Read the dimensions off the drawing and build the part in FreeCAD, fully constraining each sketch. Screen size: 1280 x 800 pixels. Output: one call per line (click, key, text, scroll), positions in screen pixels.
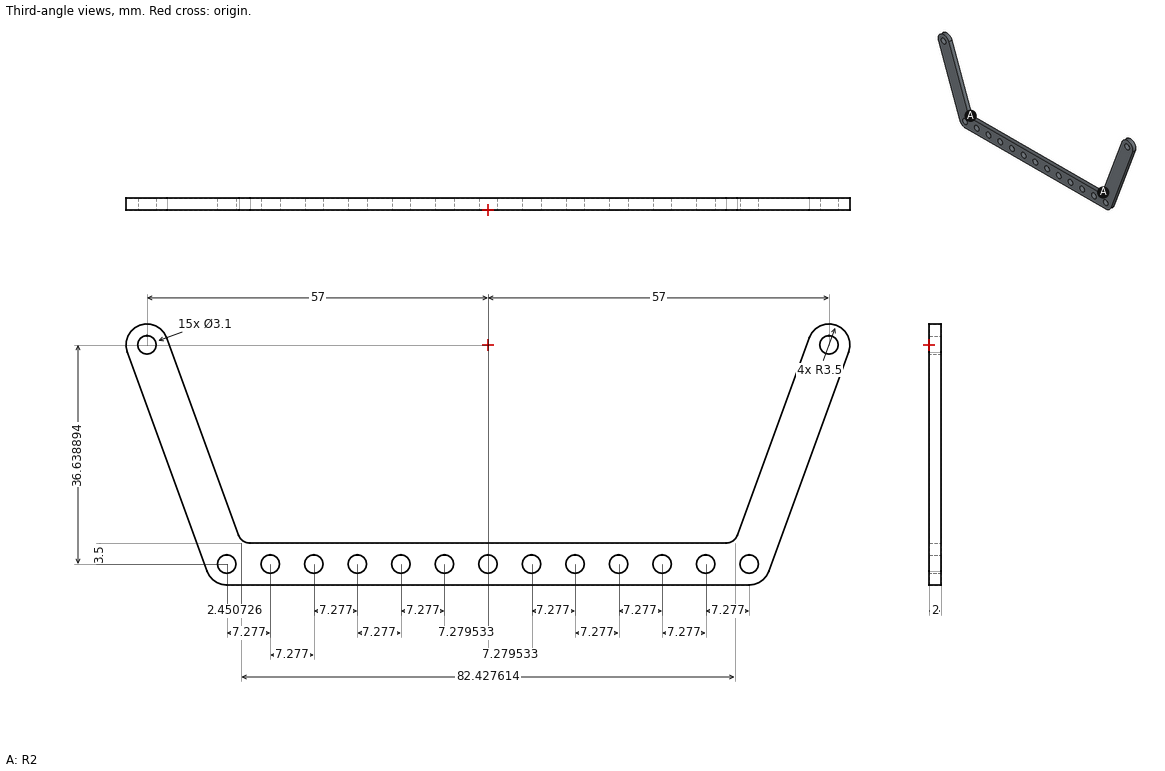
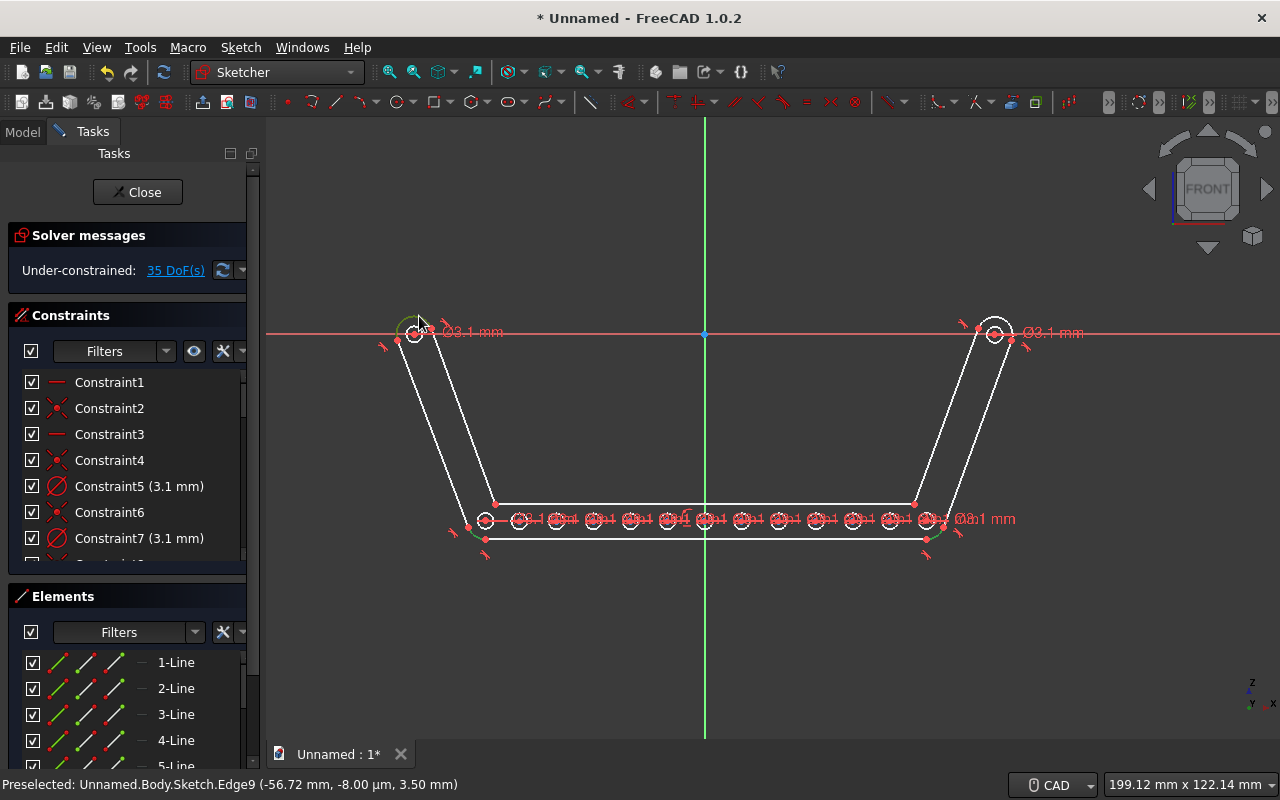
scroll(1010, 325, up, 2)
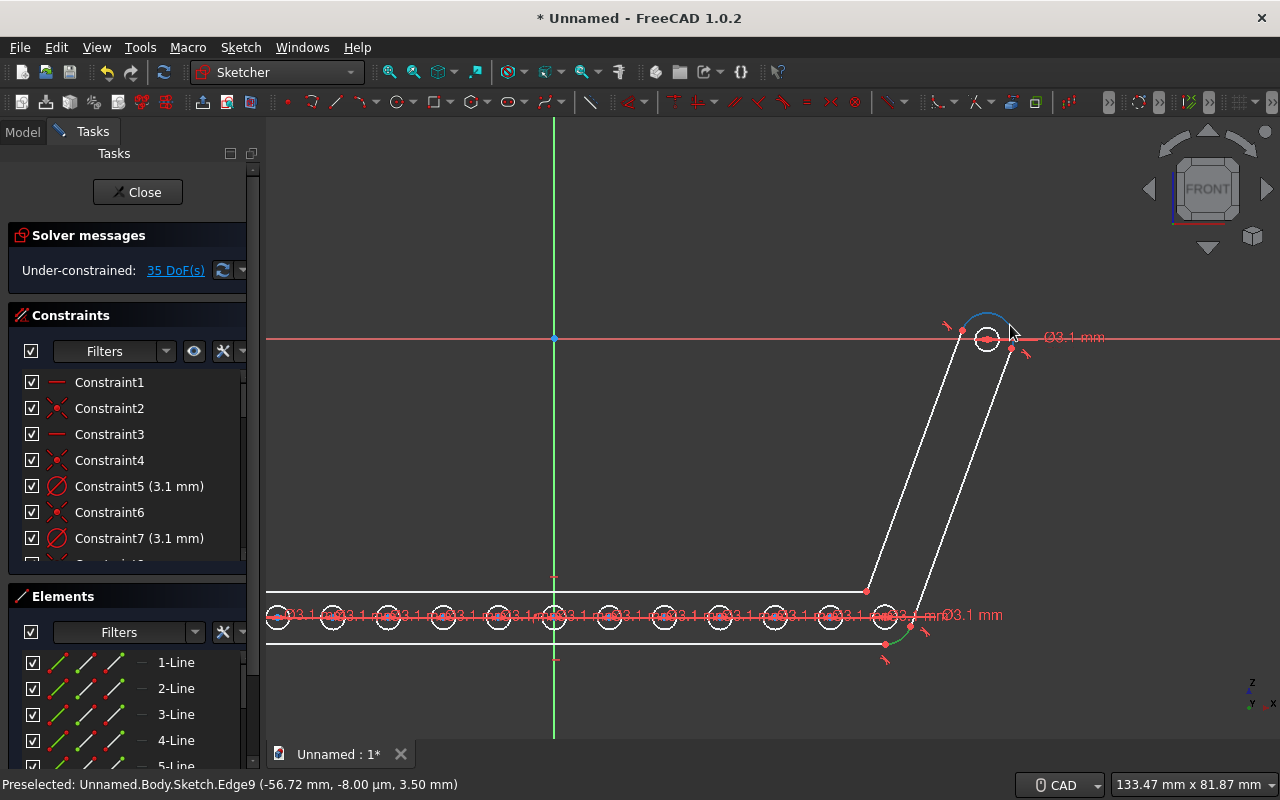
click(1009, 325)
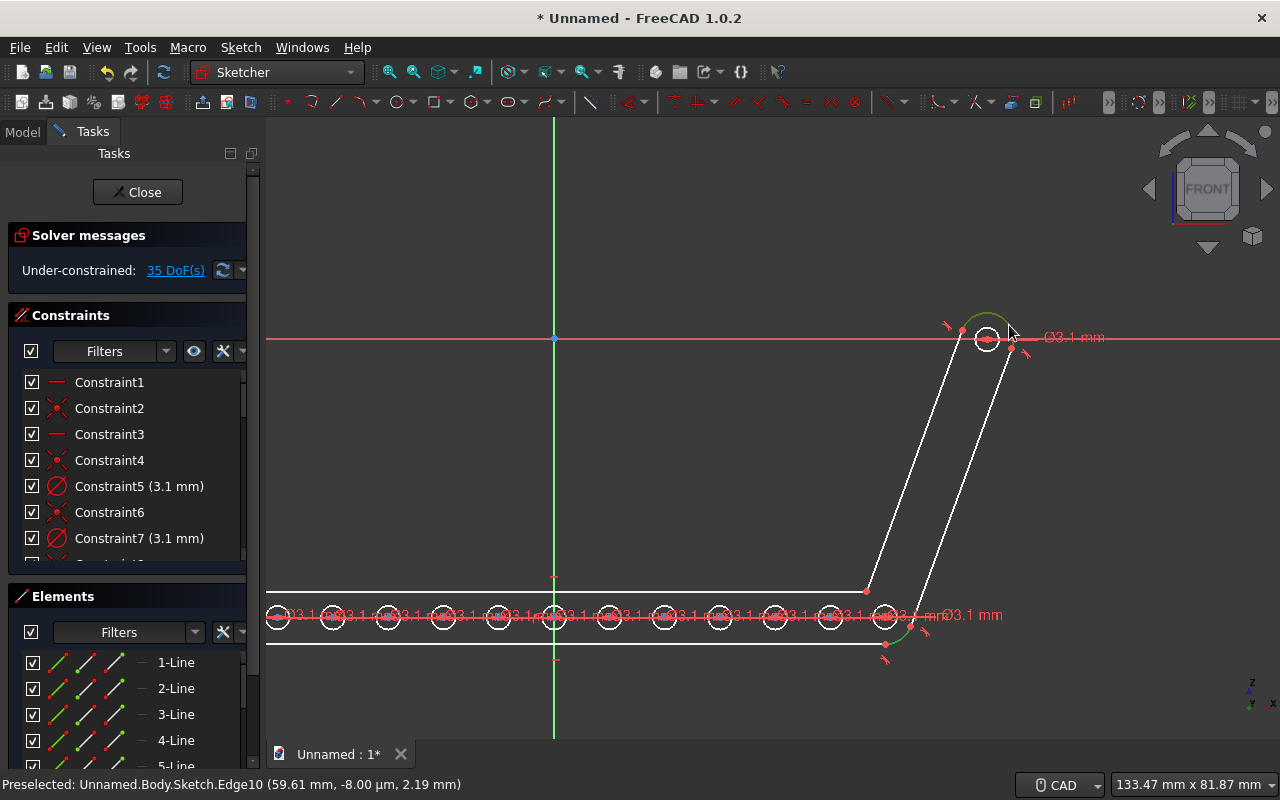
key(e)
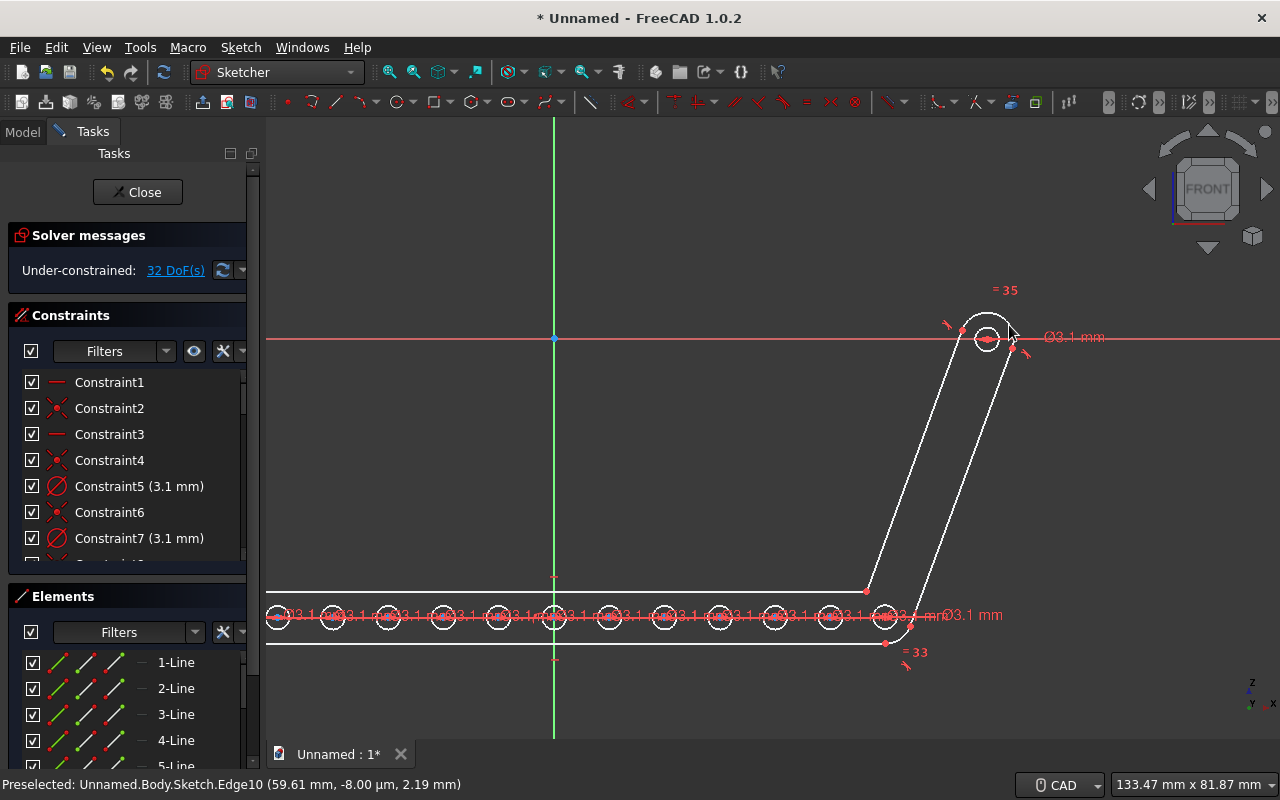
scroll(1010, 325, down, 2)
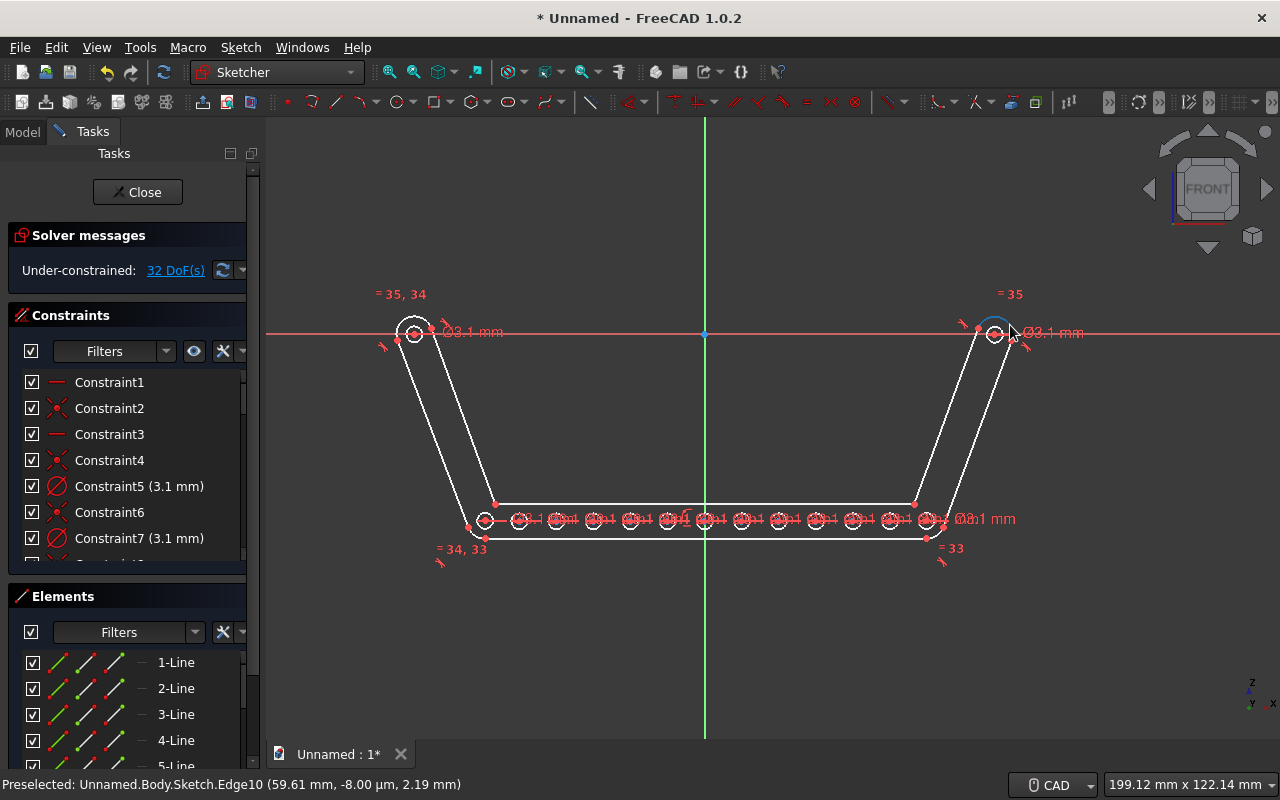
click(414, 334)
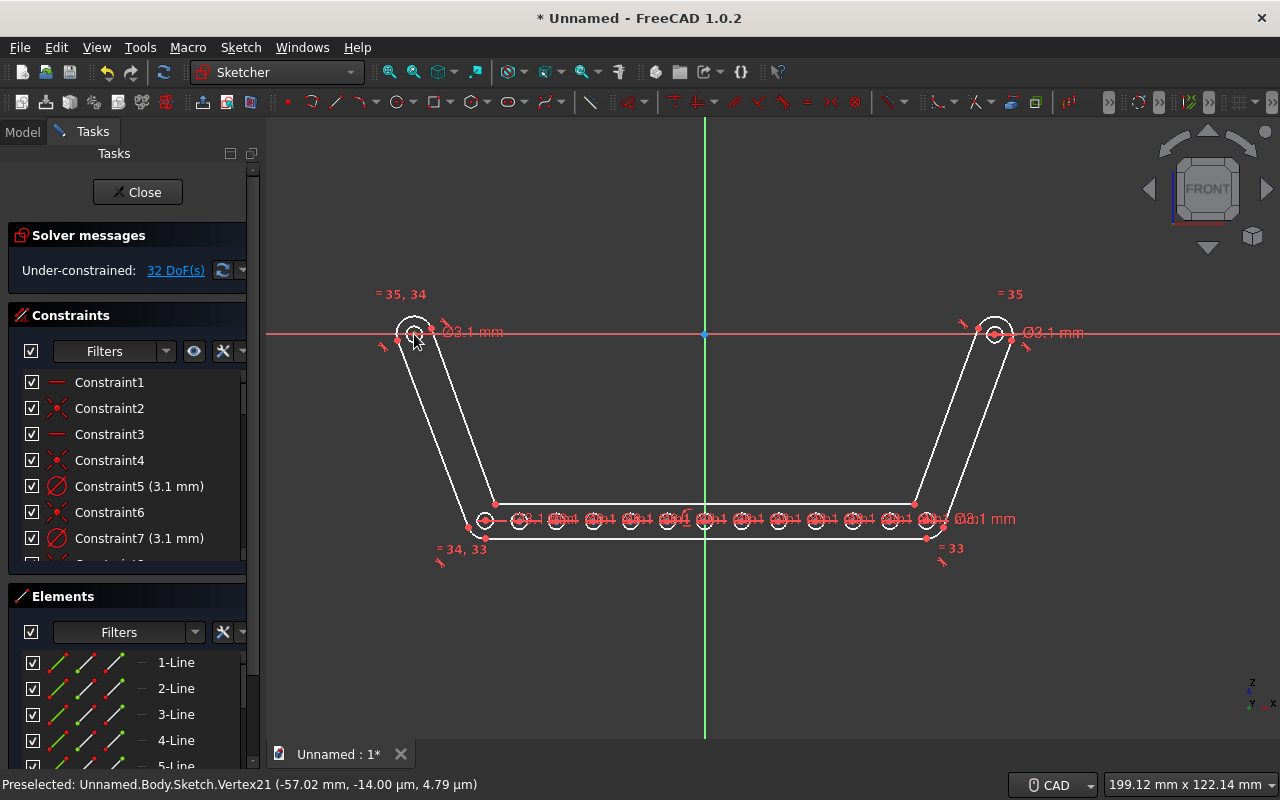
click(353, 334)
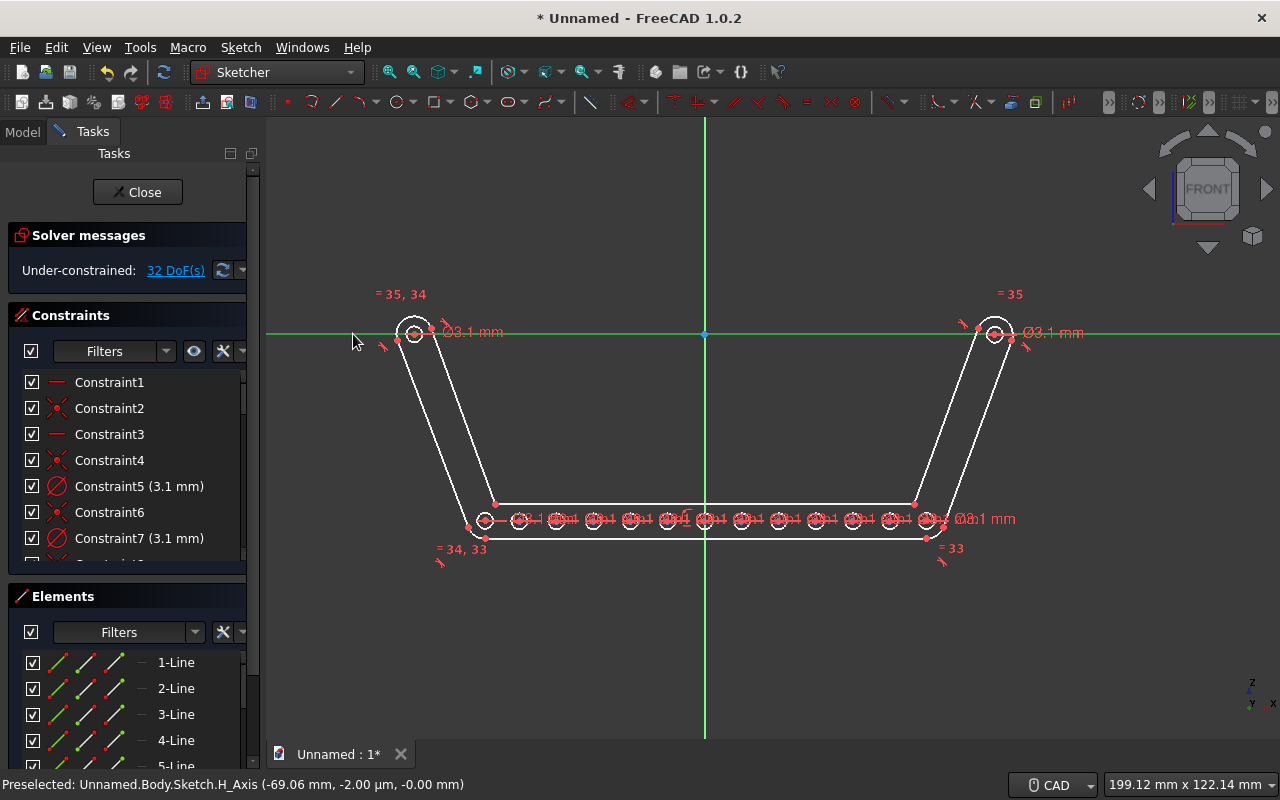
key(c)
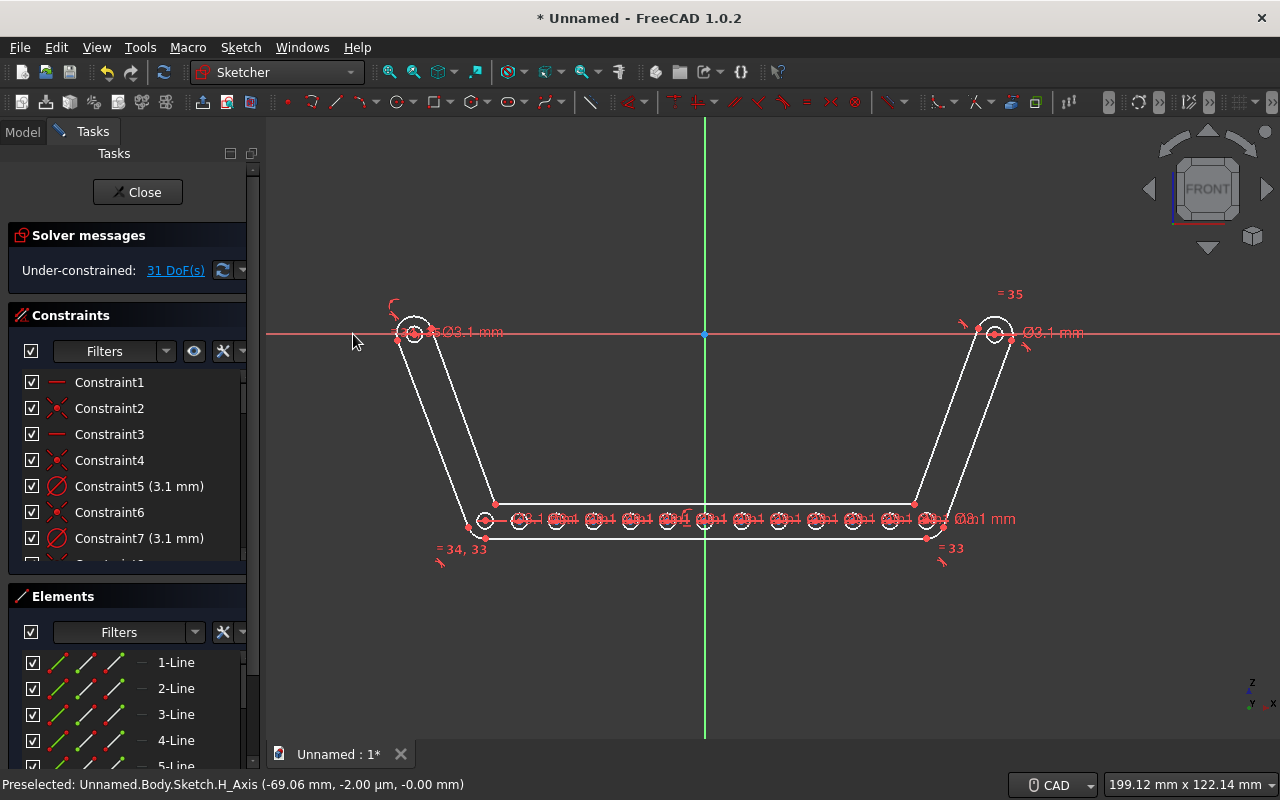
click(995, 335)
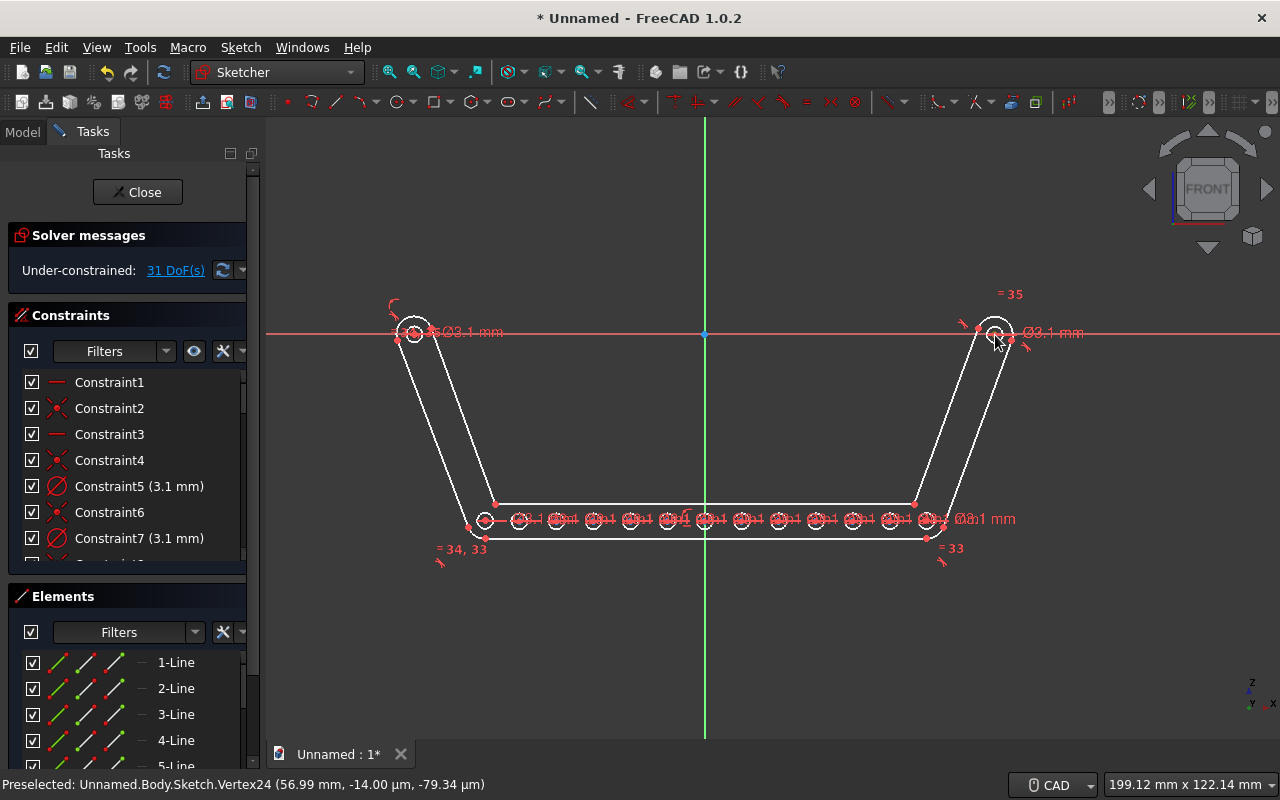
click(353, 334)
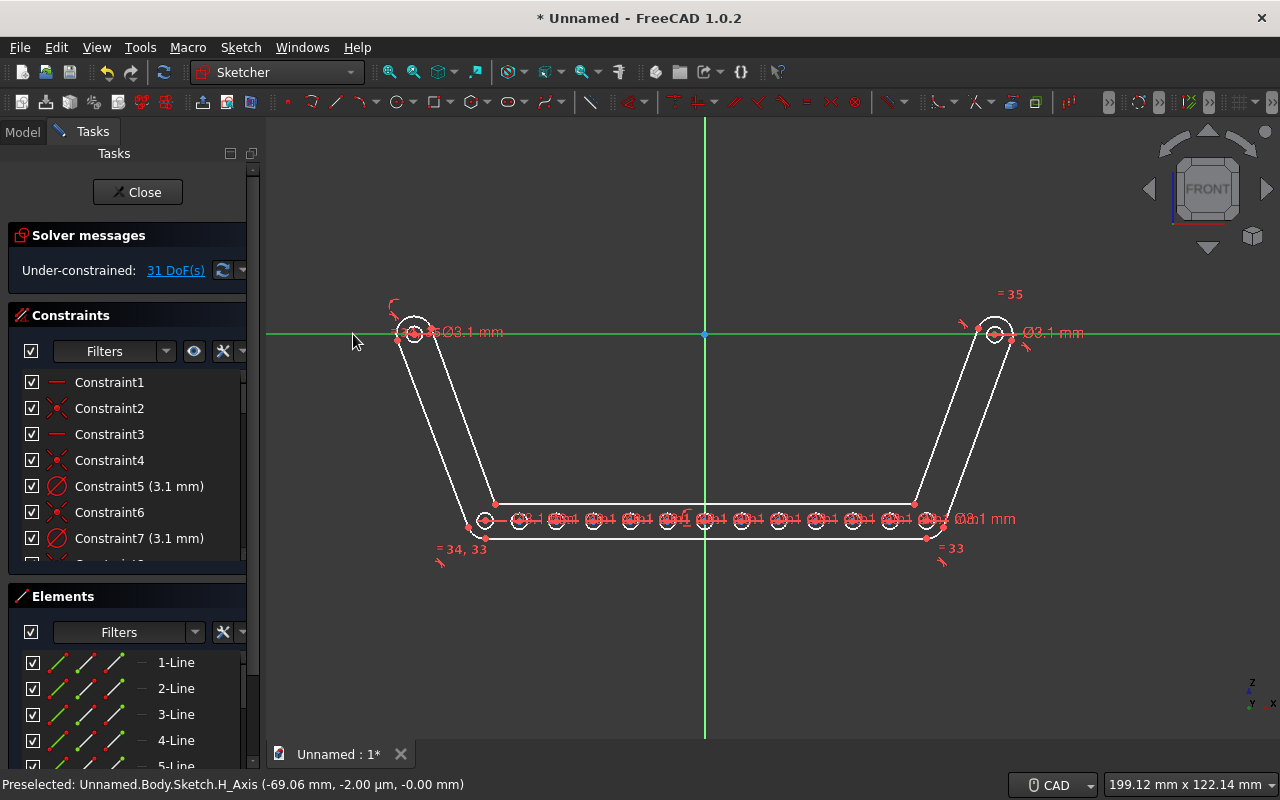
click(674, 102)